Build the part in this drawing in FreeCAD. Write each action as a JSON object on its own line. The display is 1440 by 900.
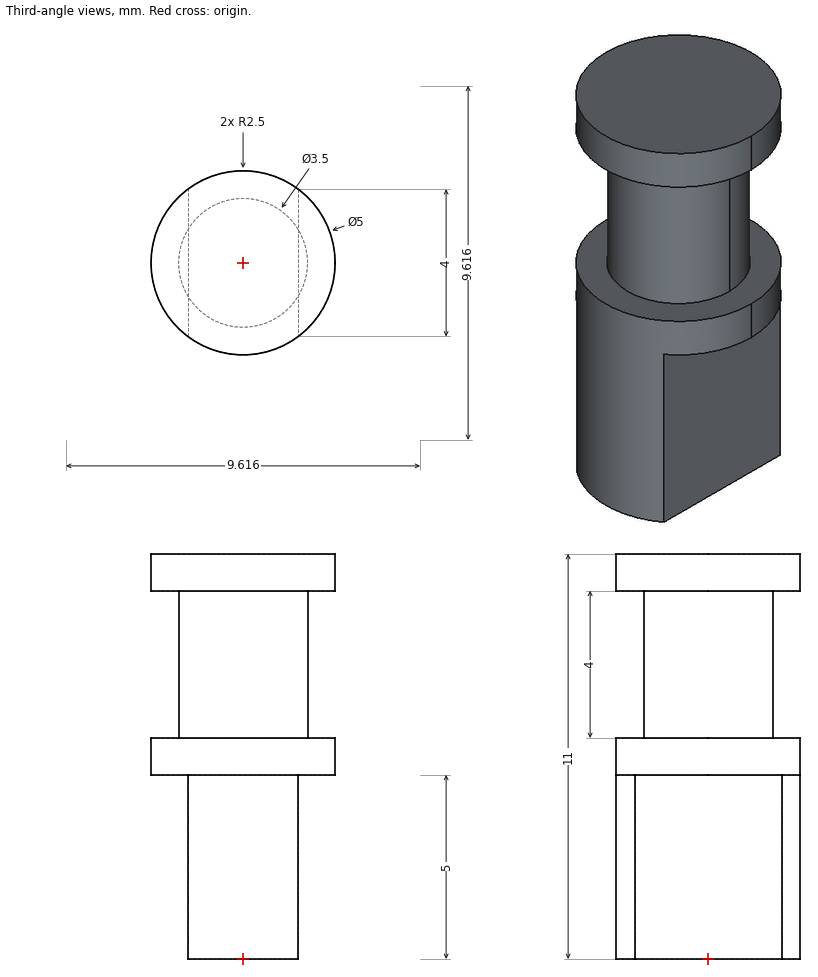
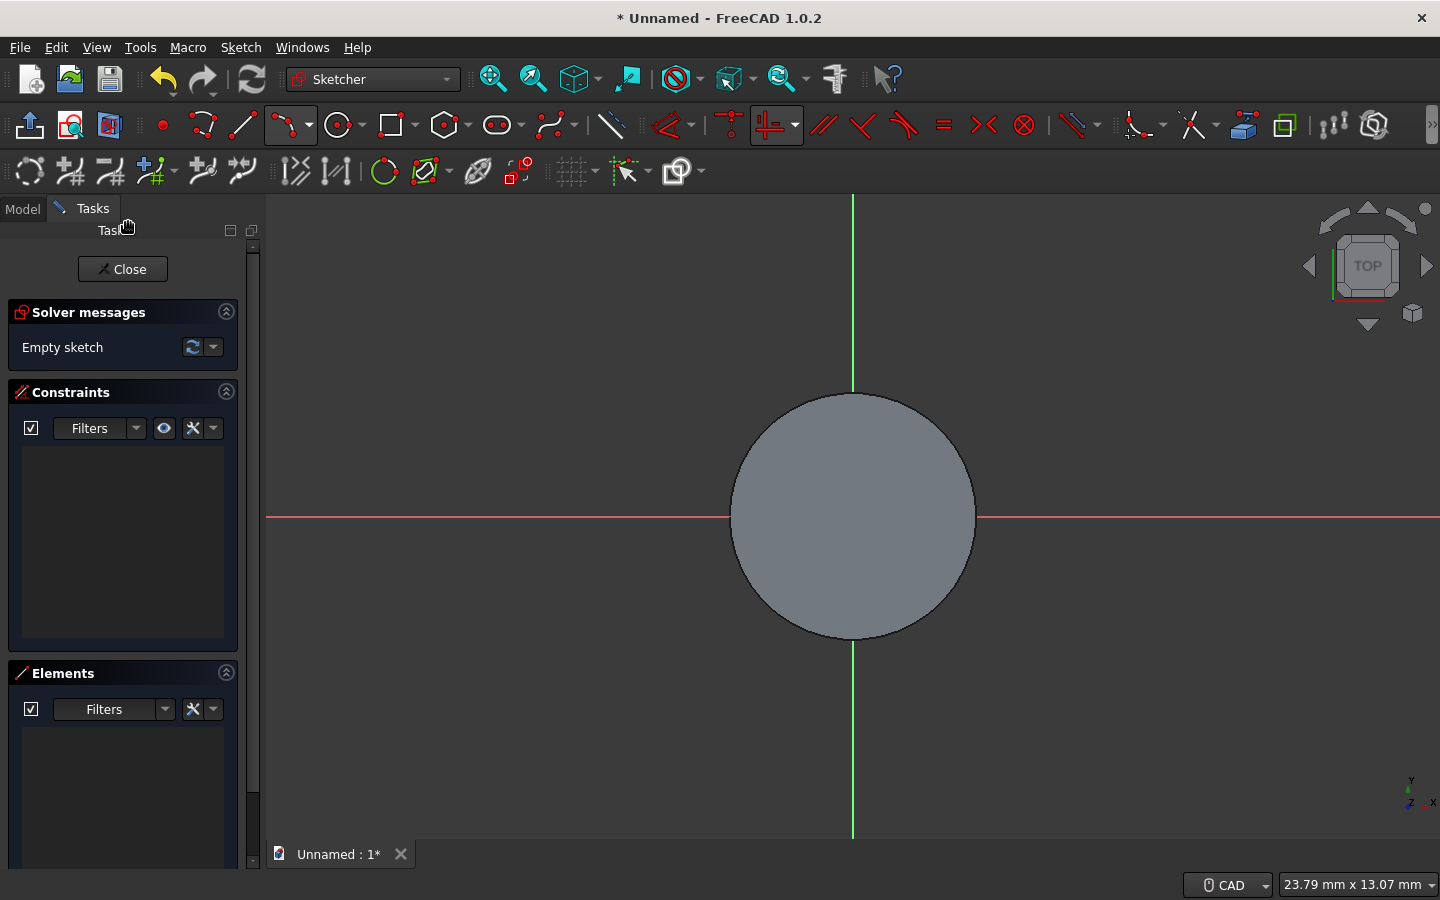
{"action": "left_click", "coordinate": [110, 126]}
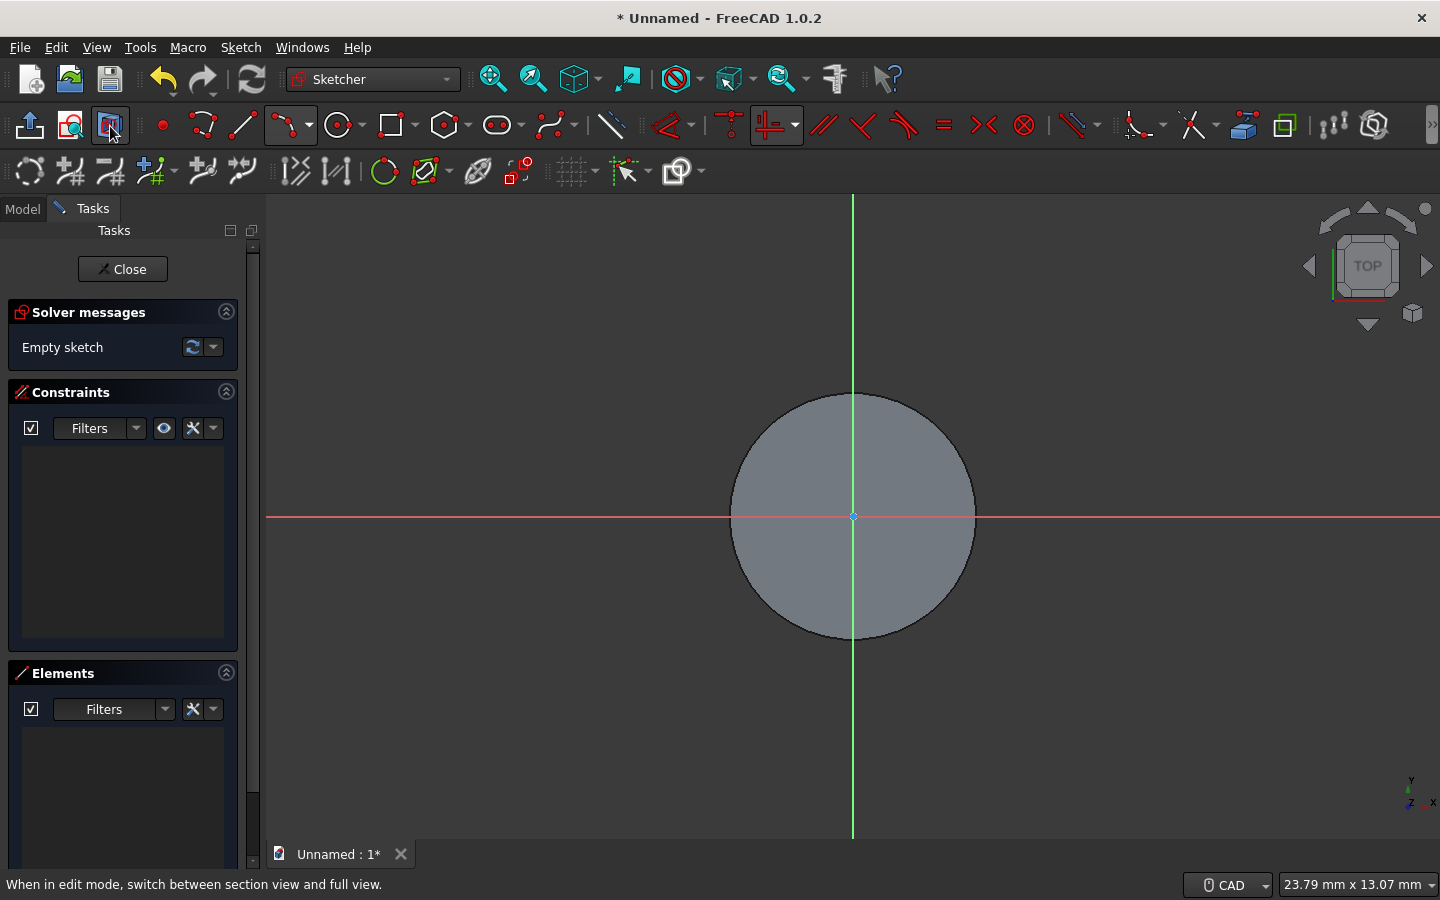
{"action": "key", "text": "g v"}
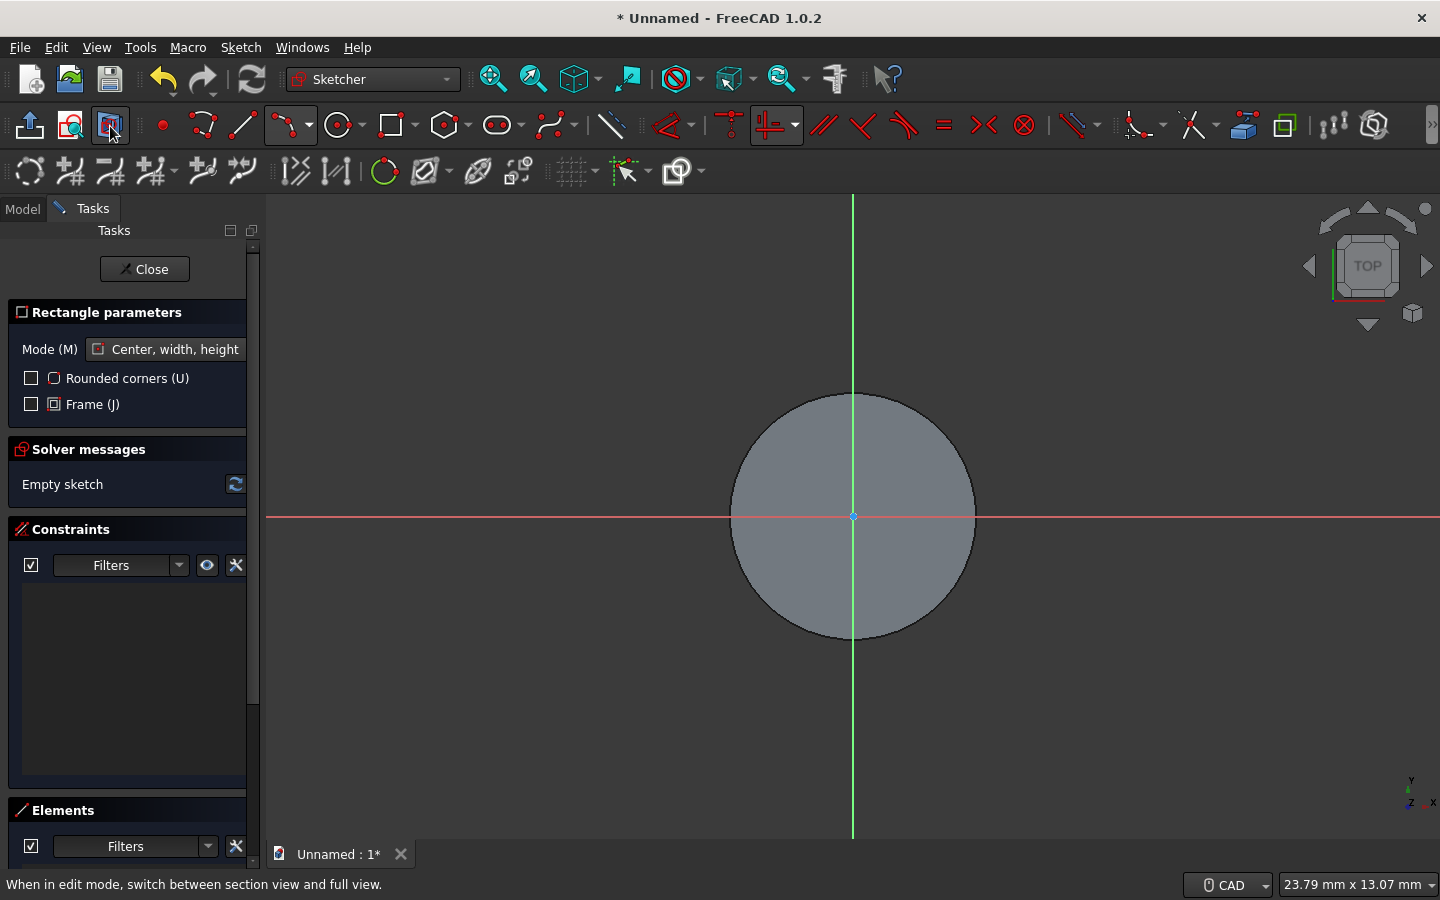
{"action": "left_click", "coordinate": [853, 516]}
{"action": "mouse_move", "coordinate": [1090, 279]}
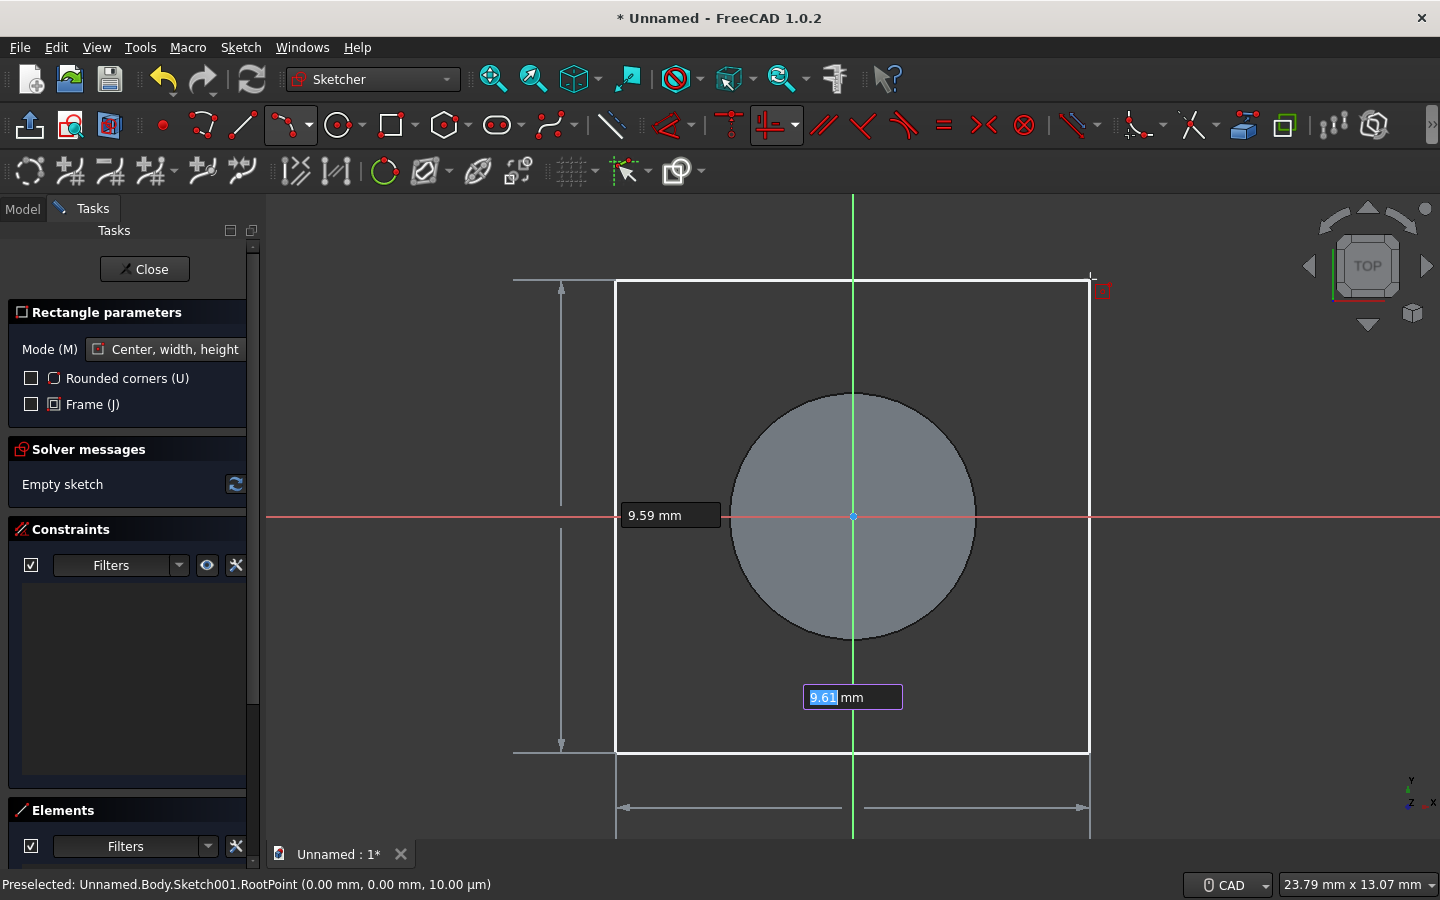
{"action": "type", "text": "9.616"}
{"action": "key", "text": "Tab"}
{"action": "type", "text": "9.616"}
{"action": "key", "text": "Return"}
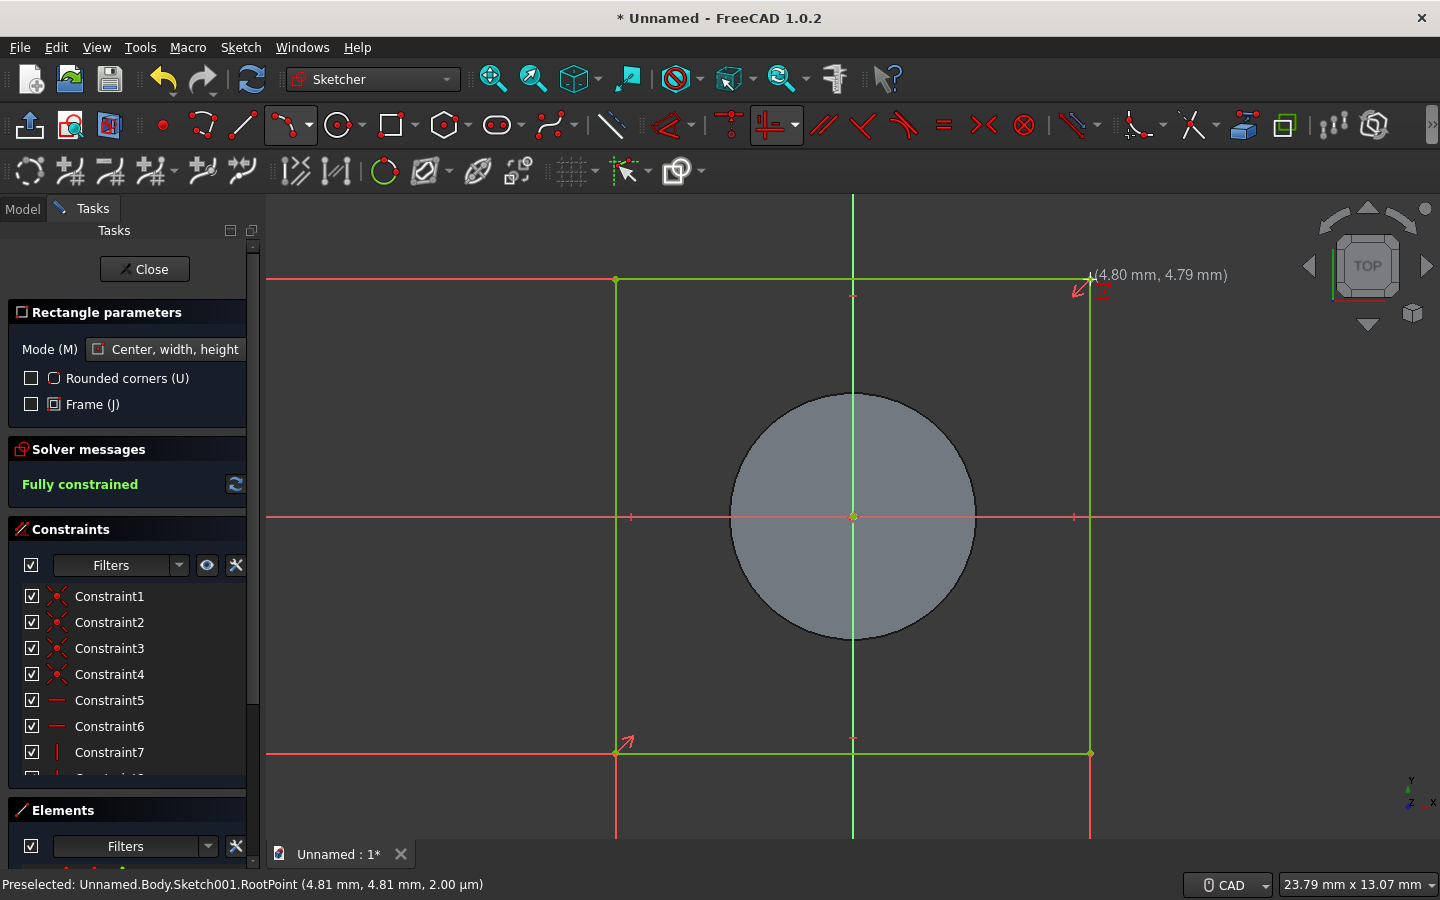
{"action": "key", "text": "g l"}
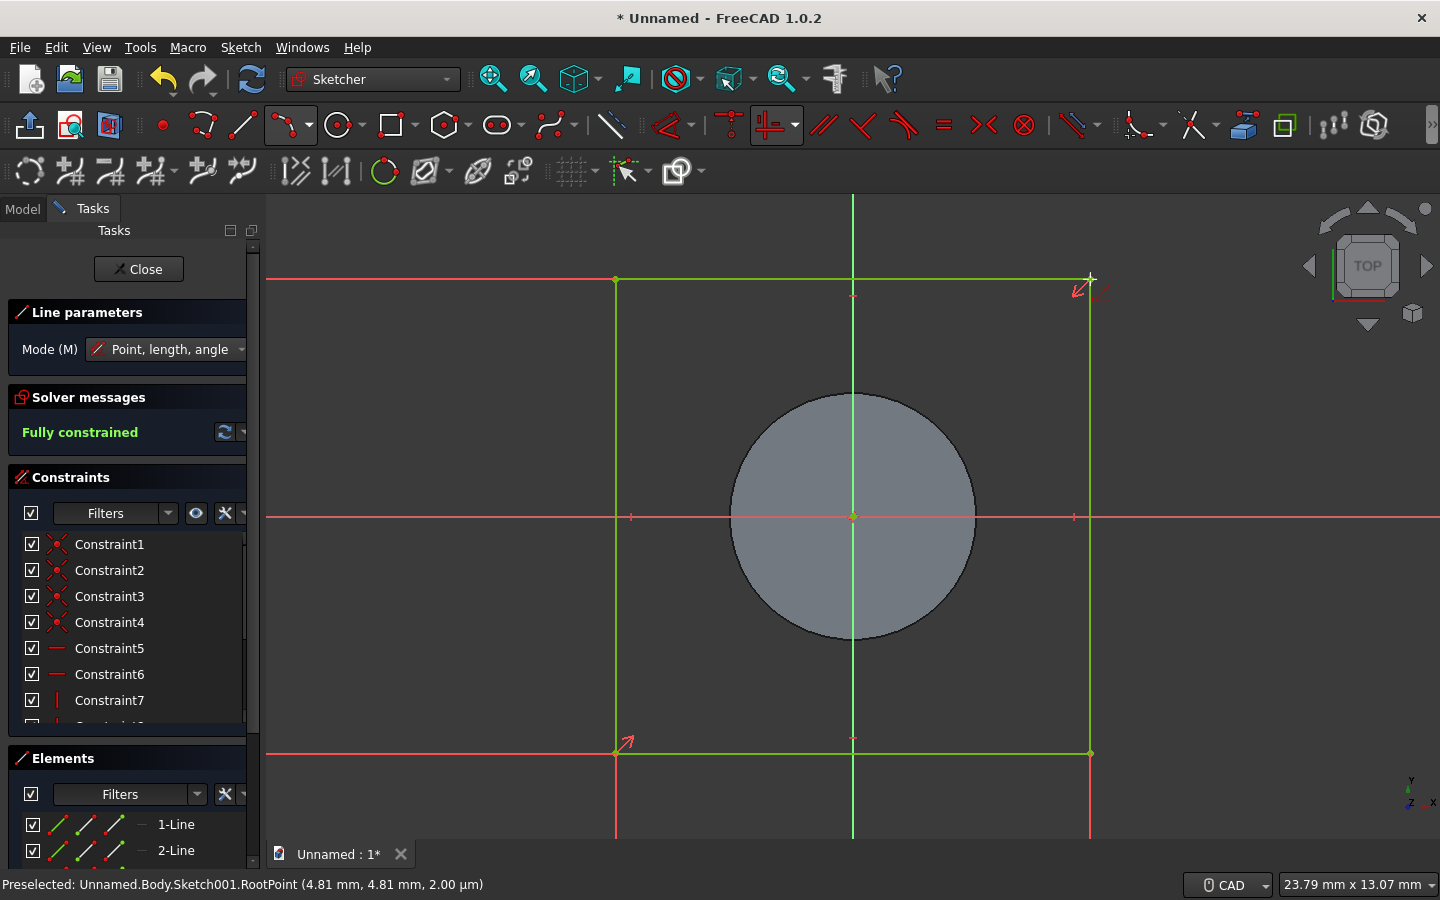
{"action": "left_click", "coordinate": [927, 615]}
{"action": "left_click", "coordinate": [927, 418]}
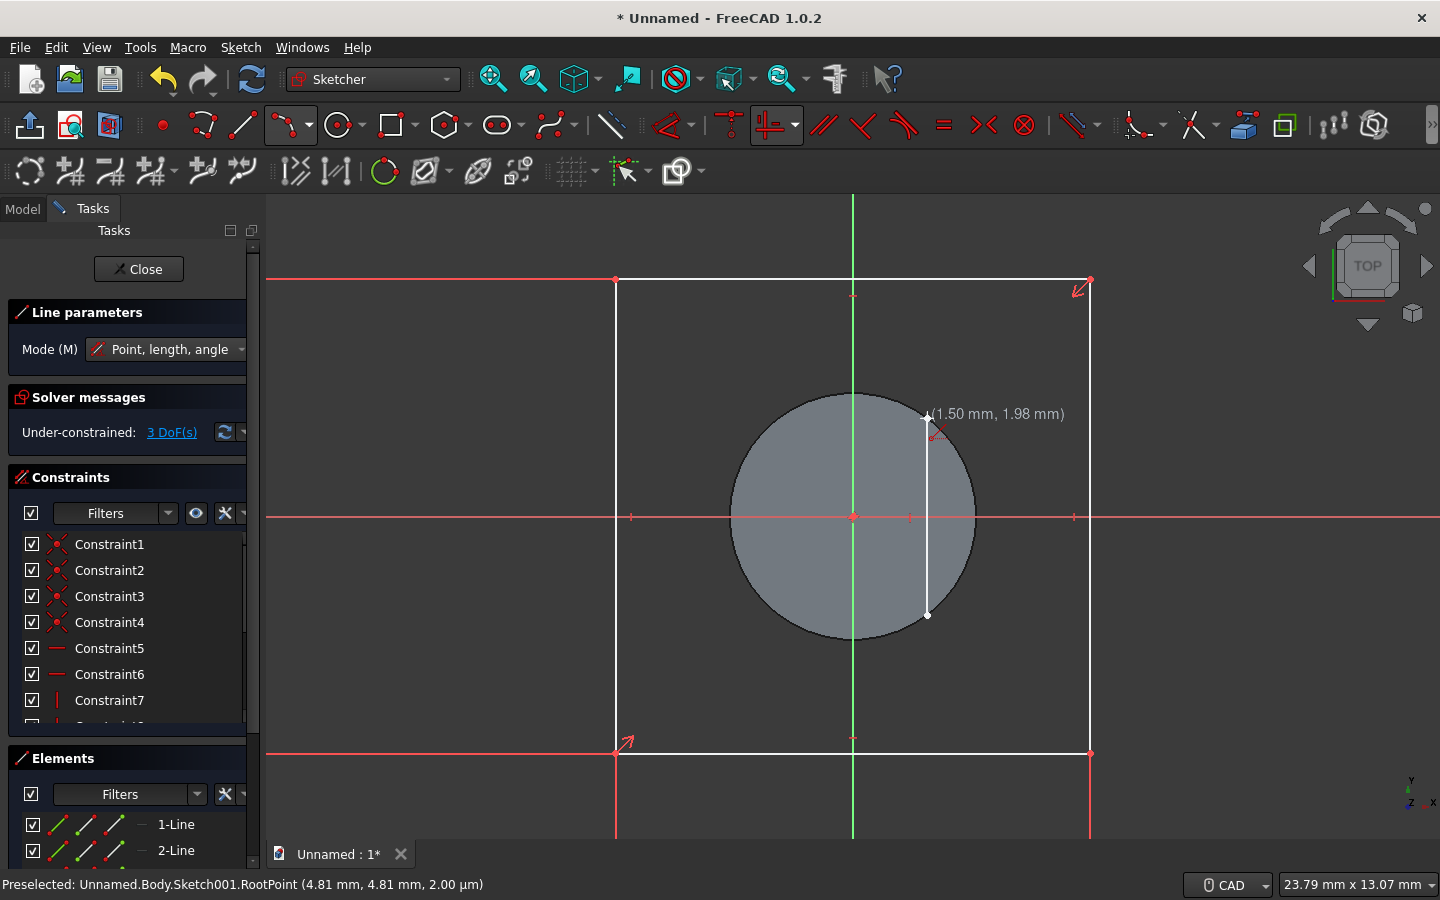
{"action": "left_click", "coordinate": [779, 418]}
{"action": "left_click", "coordinate": [779, 615]}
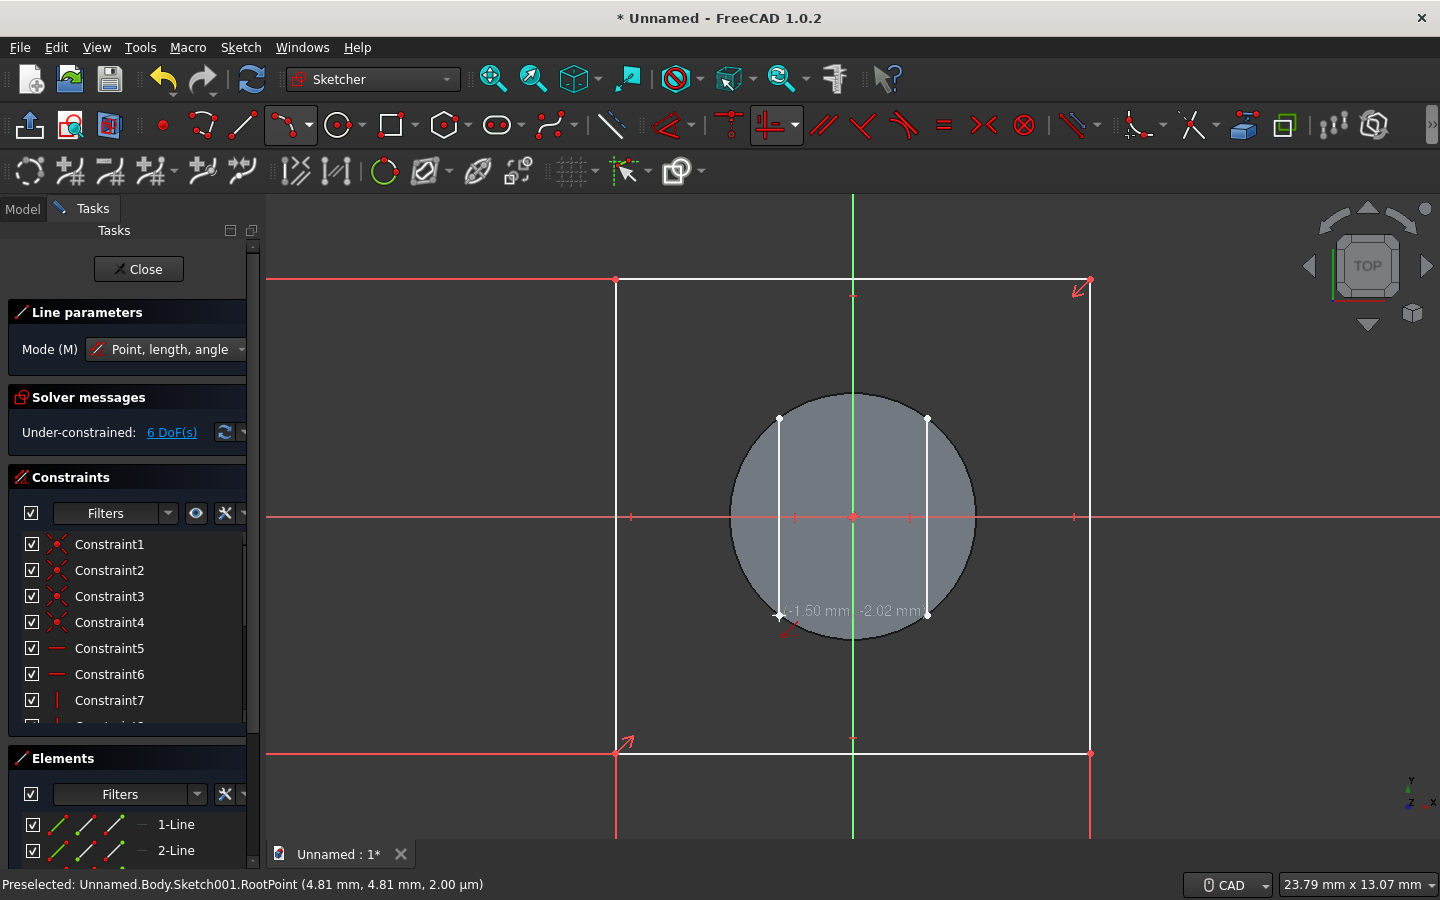
{"action": "key", "text": "g 3 a"}